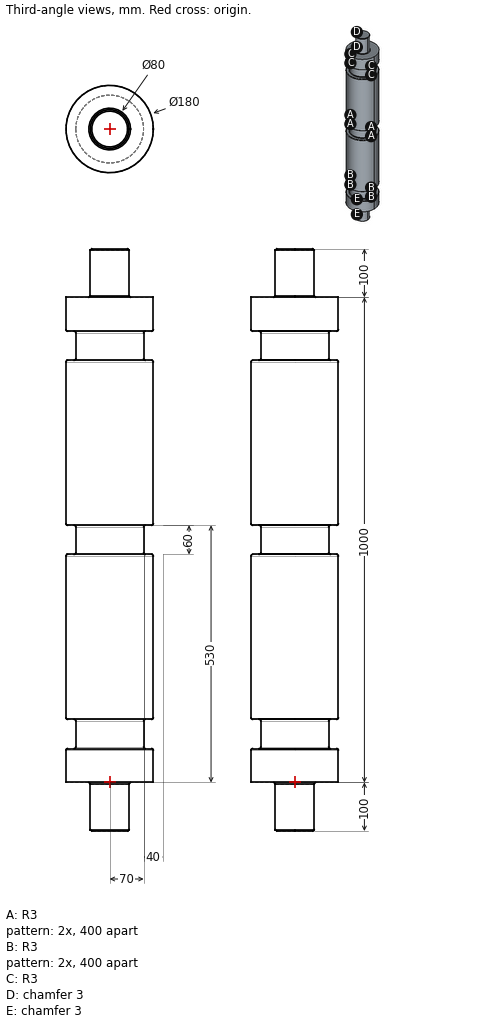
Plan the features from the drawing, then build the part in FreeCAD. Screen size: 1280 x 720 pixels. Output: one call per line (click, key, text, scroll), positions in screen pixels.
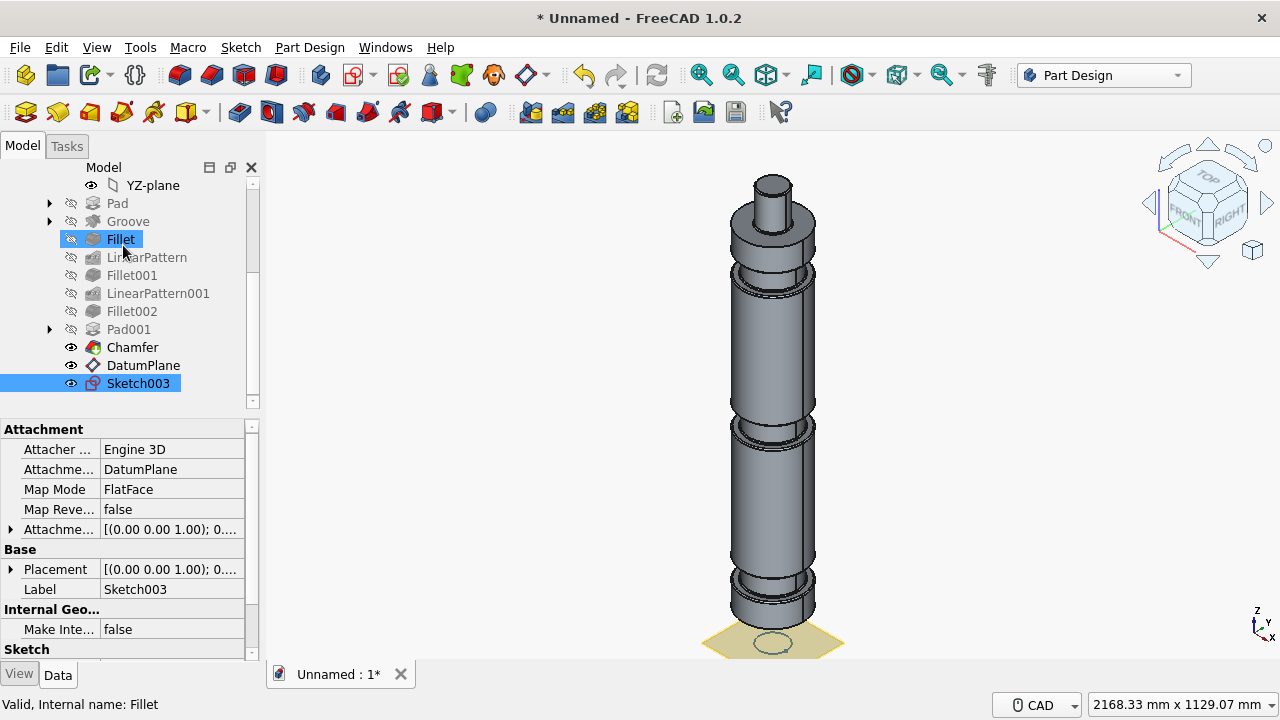
click(26, 112)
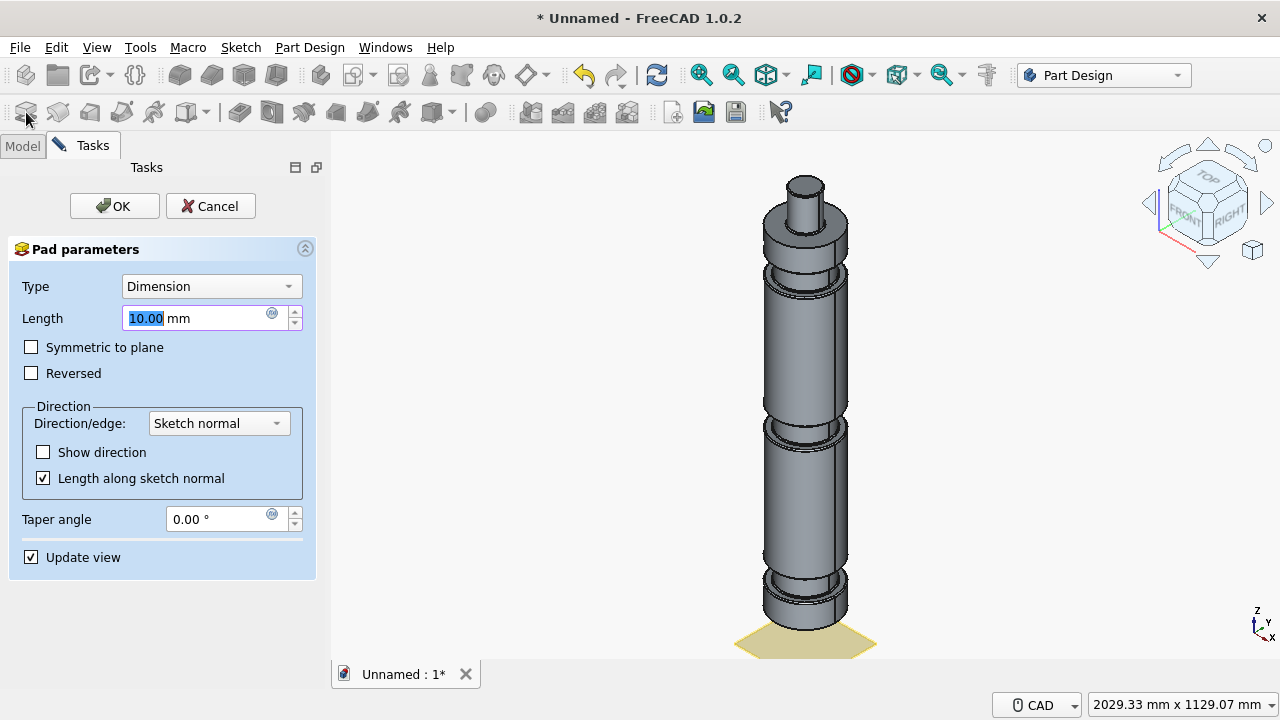
text(100)
key(Tab)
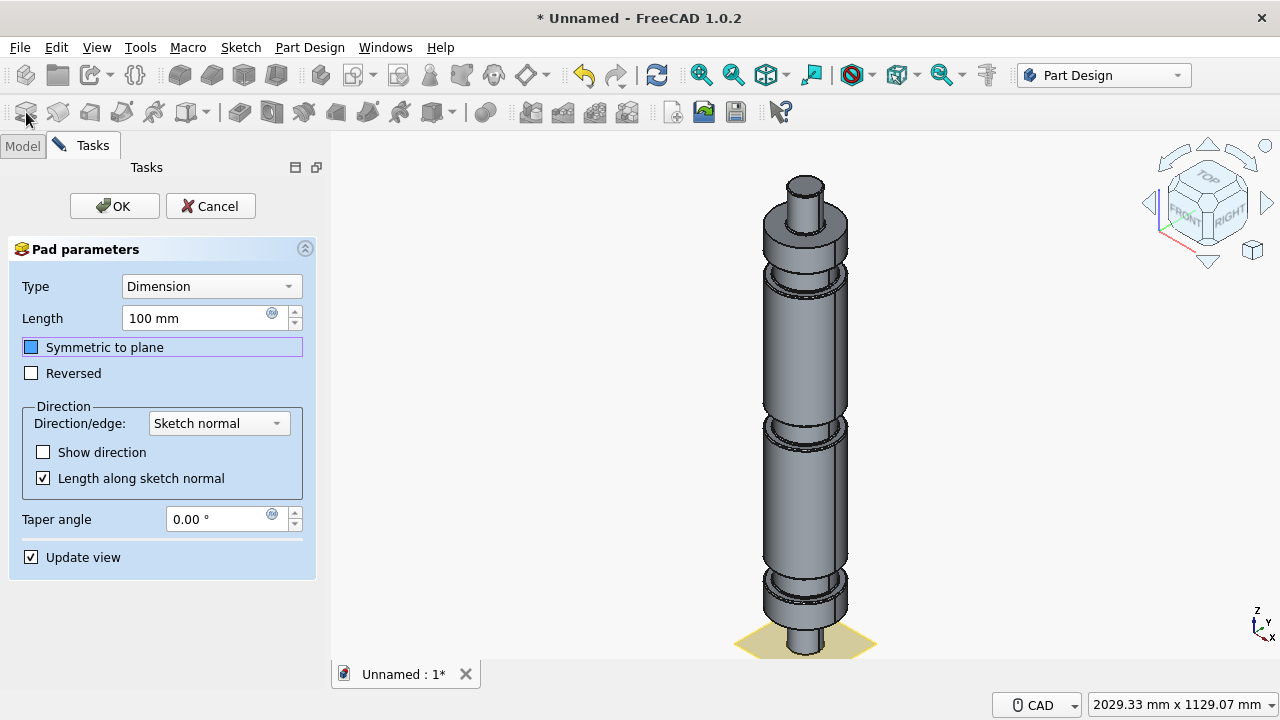
click(115, 206)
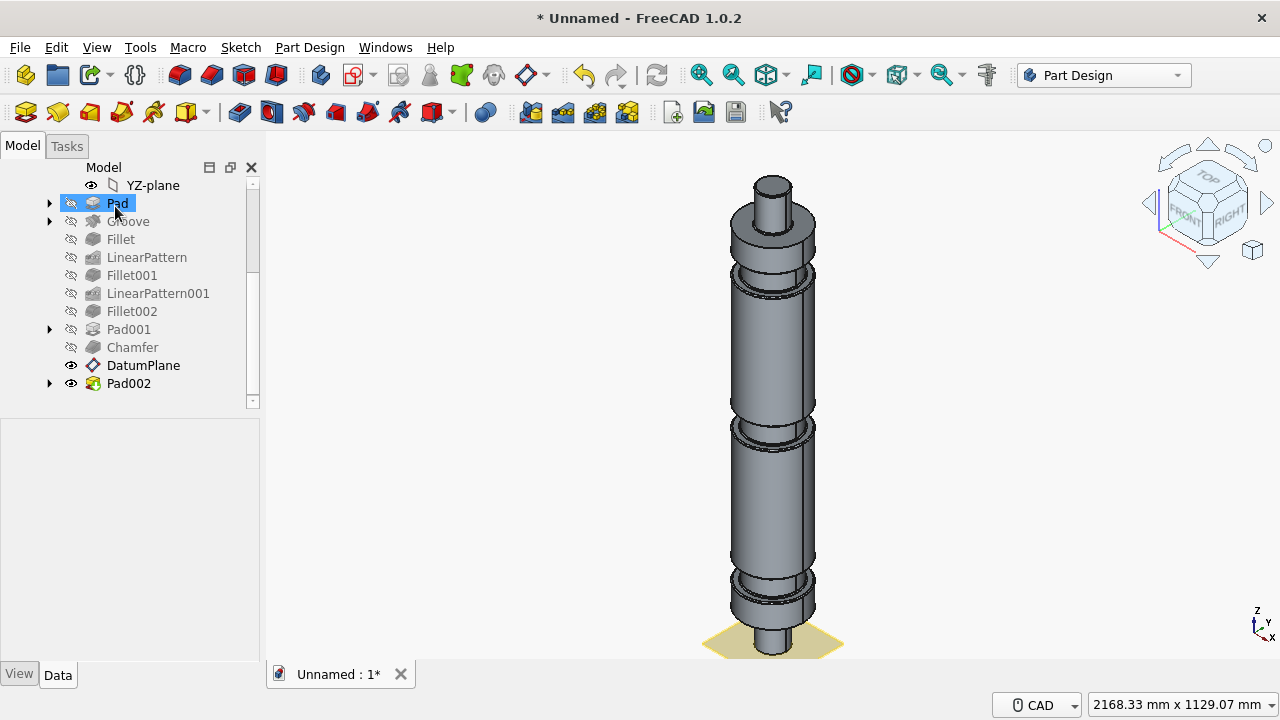
click(116, 365)
key(space)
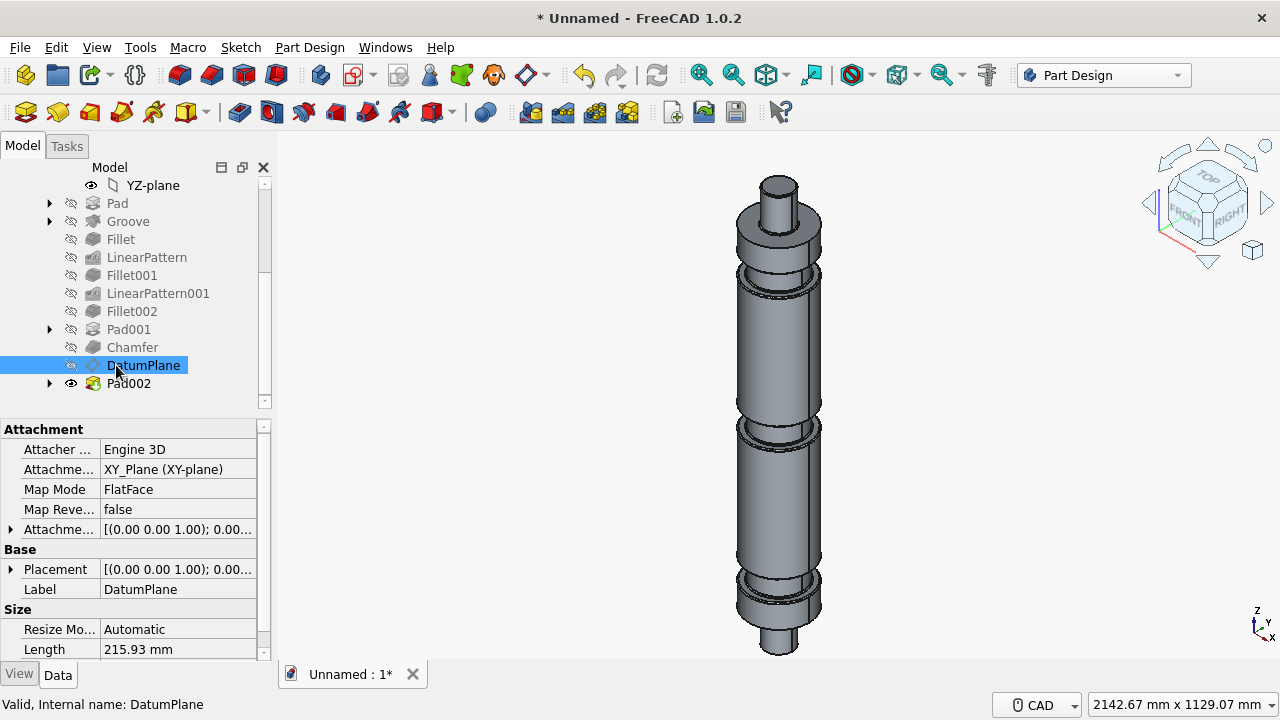
click(702, 76)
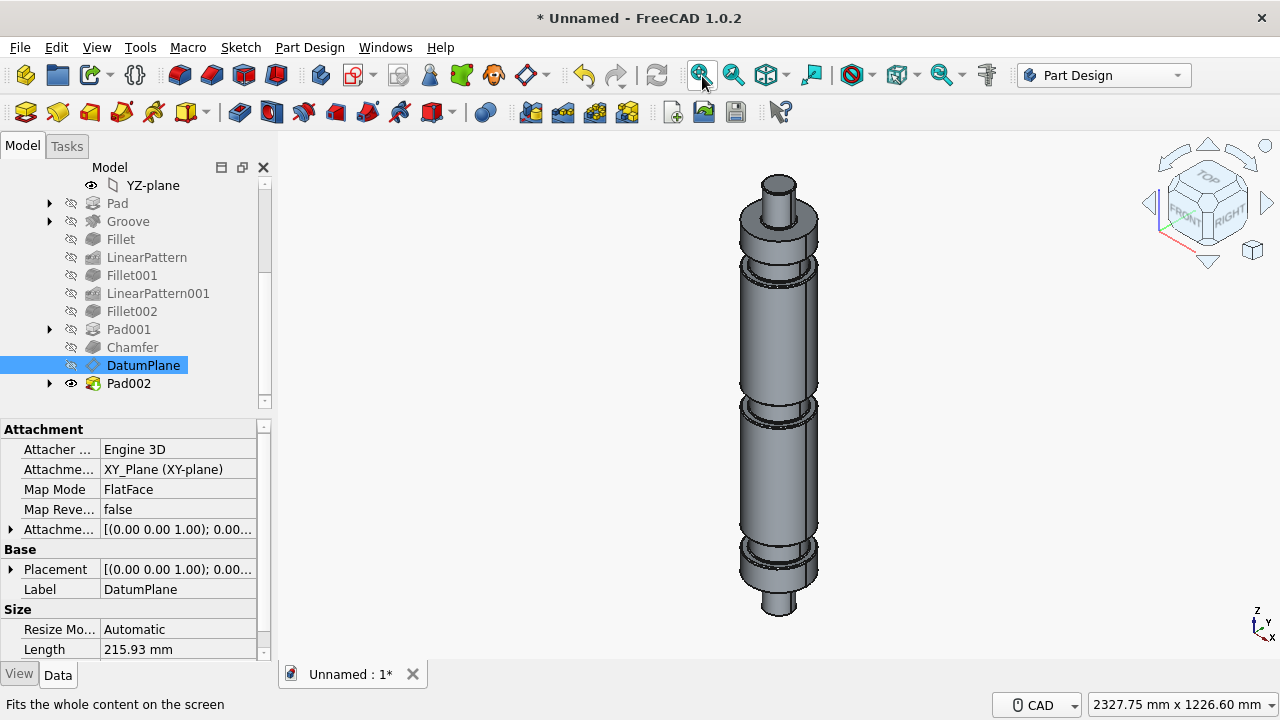
click(771, 614)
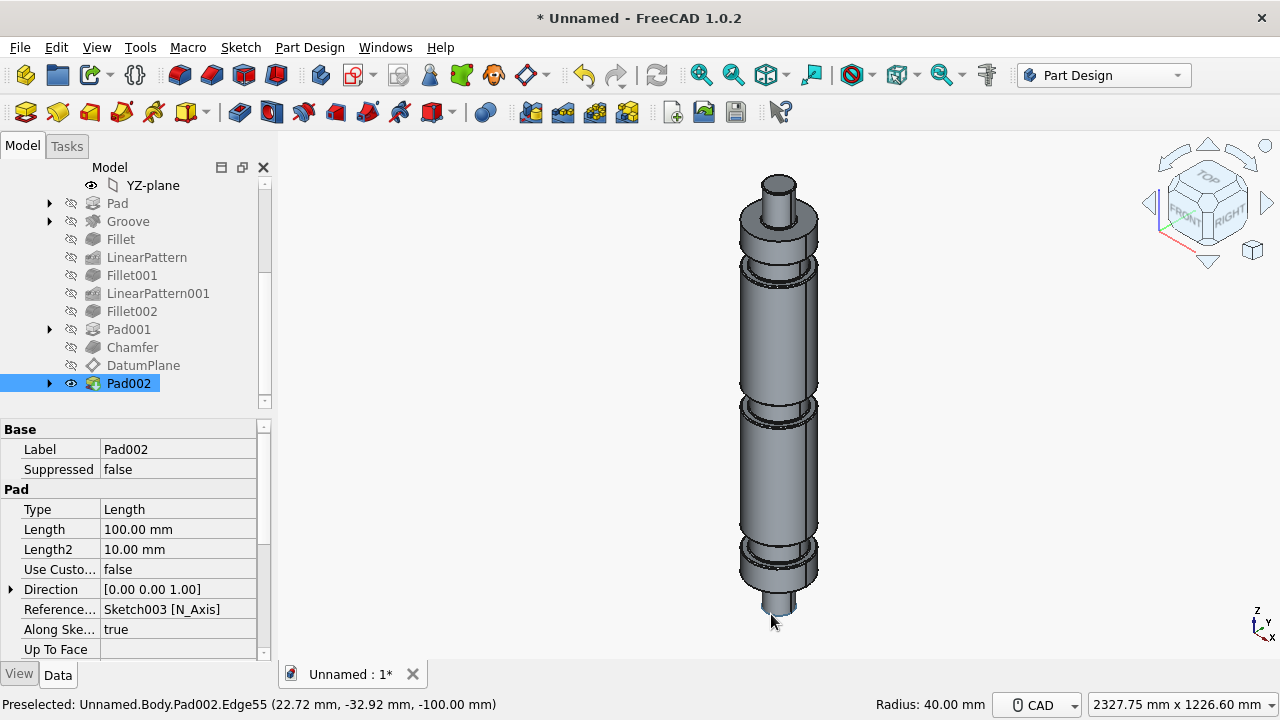
key(2)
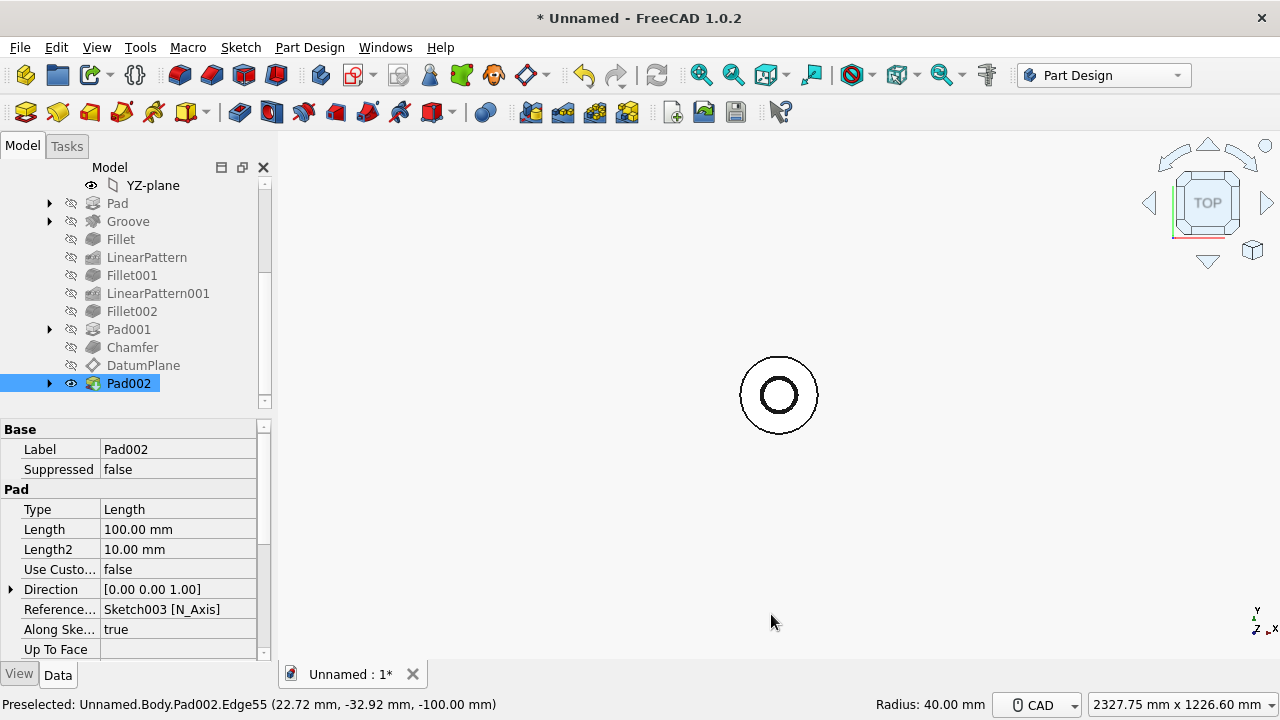
click(702, 76)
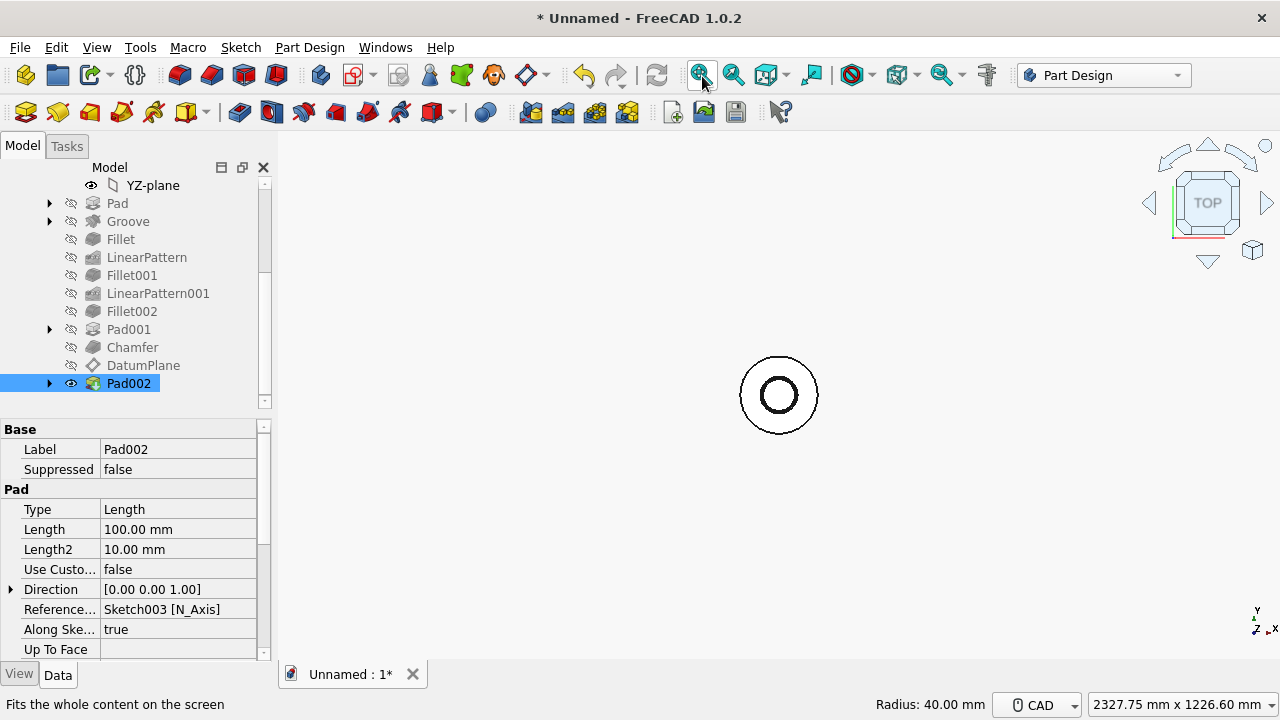
key(0)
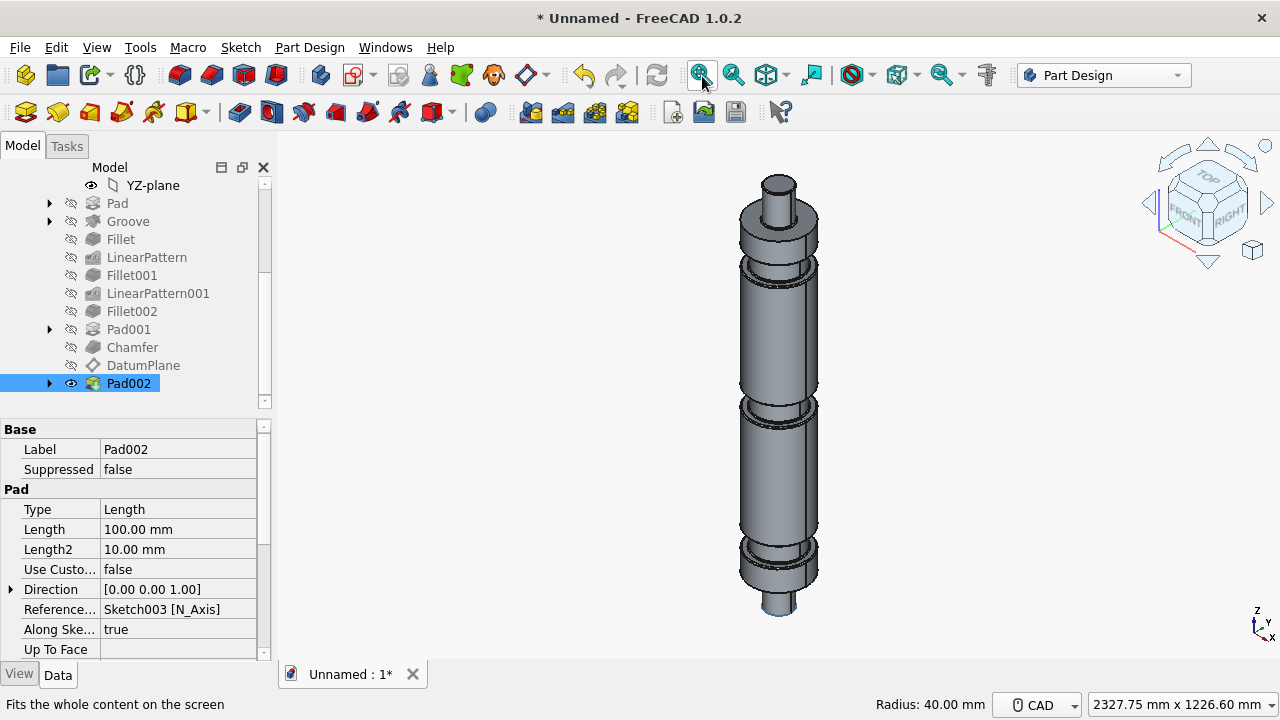
key(1)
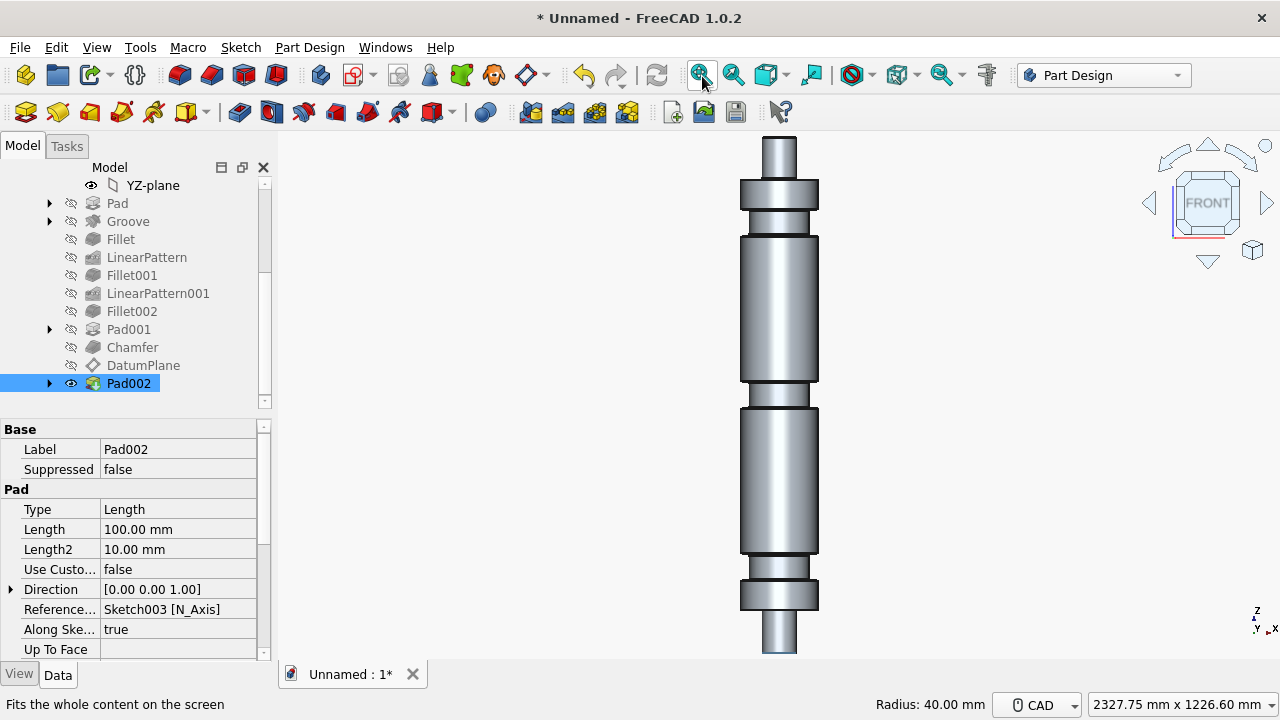
key(3)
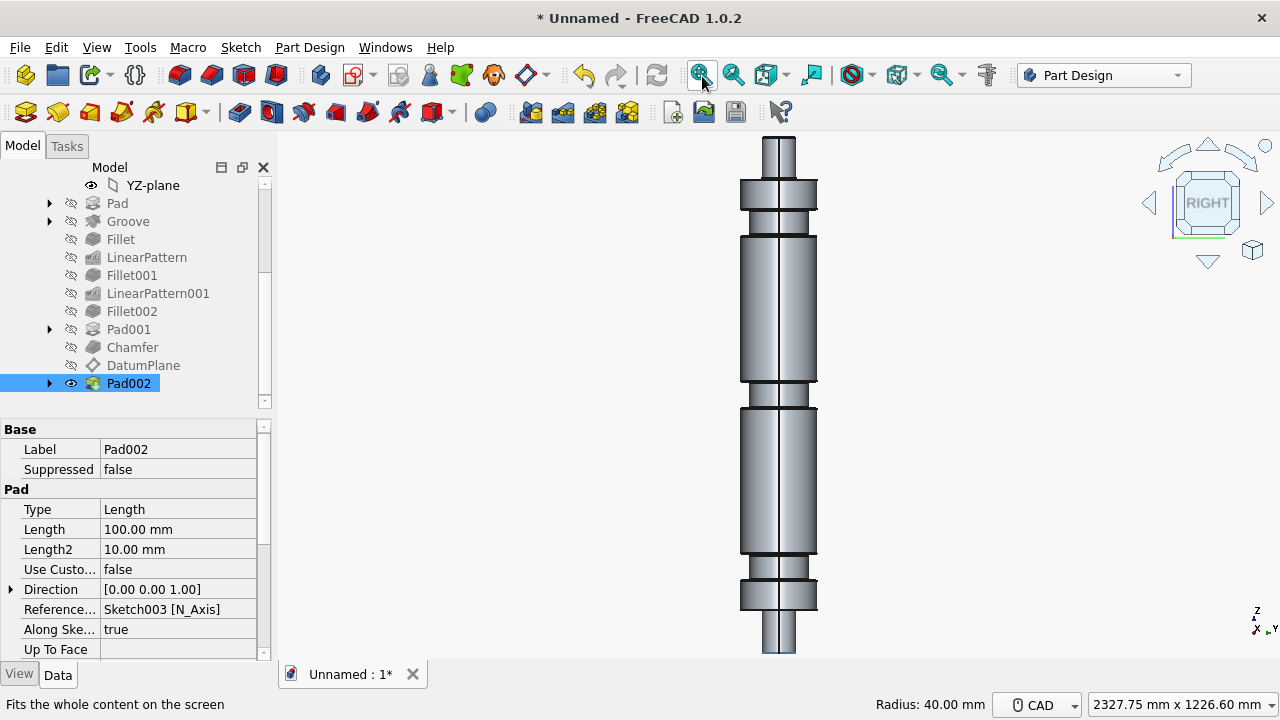
key(5)